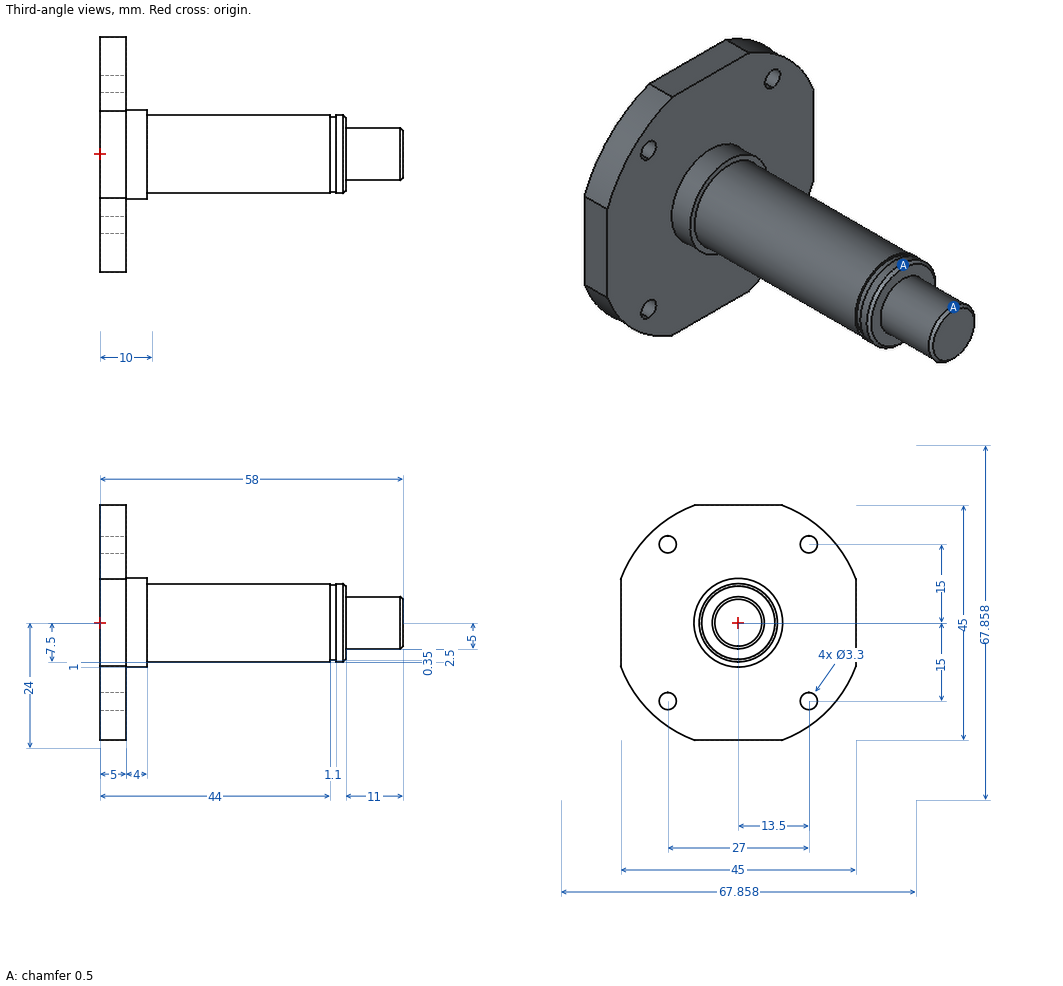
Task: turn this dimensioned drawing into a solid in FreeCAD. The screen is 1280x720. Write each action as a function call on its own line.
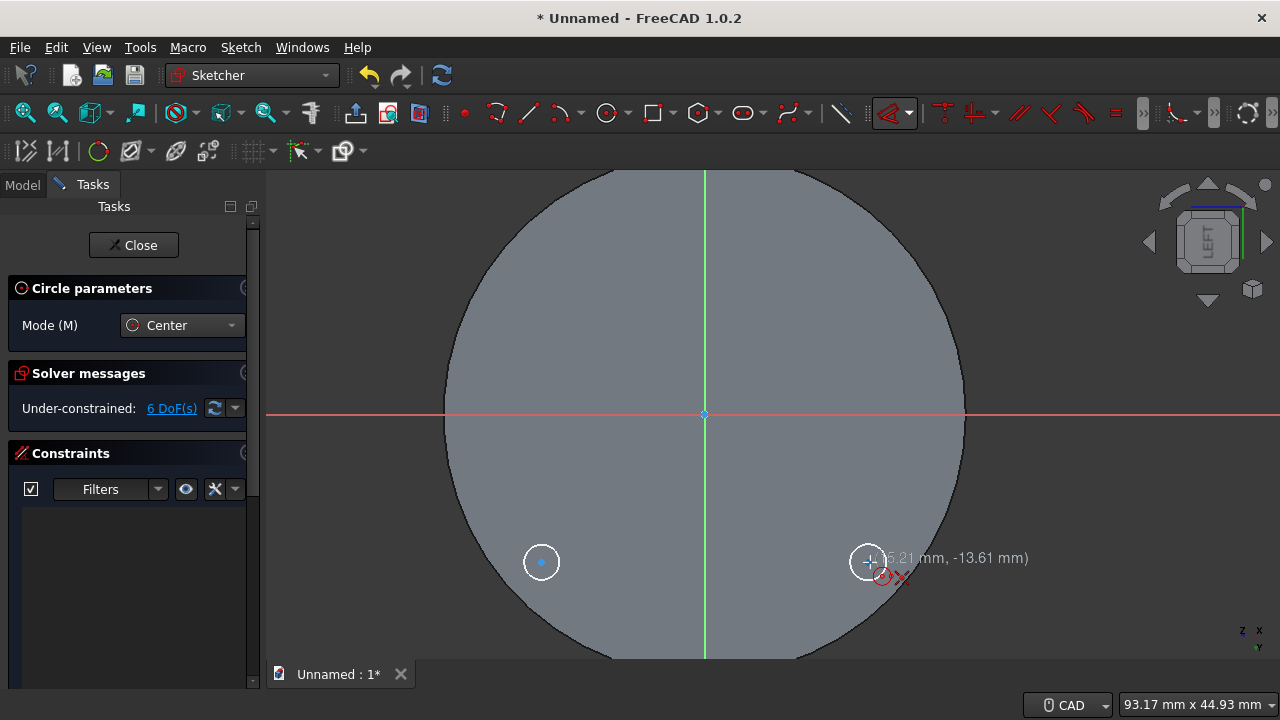
scroll(868, 268, up, 2)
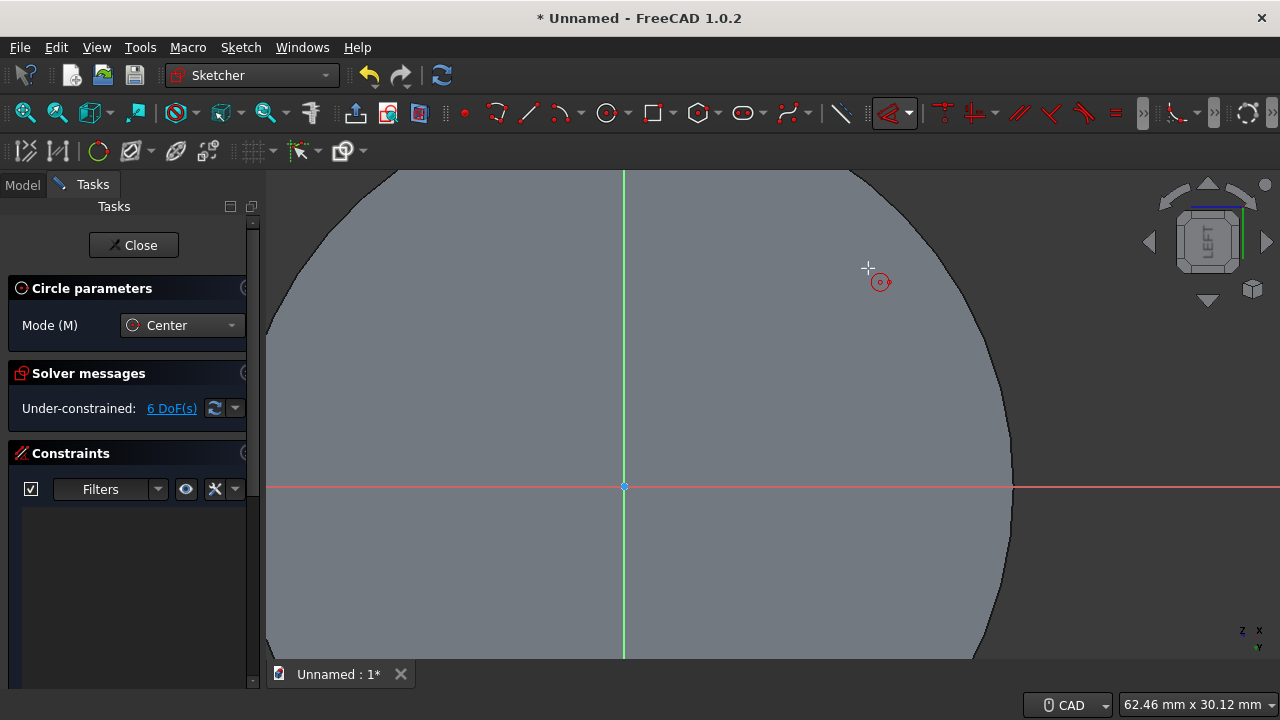
click(868, 268)
click(887, 249)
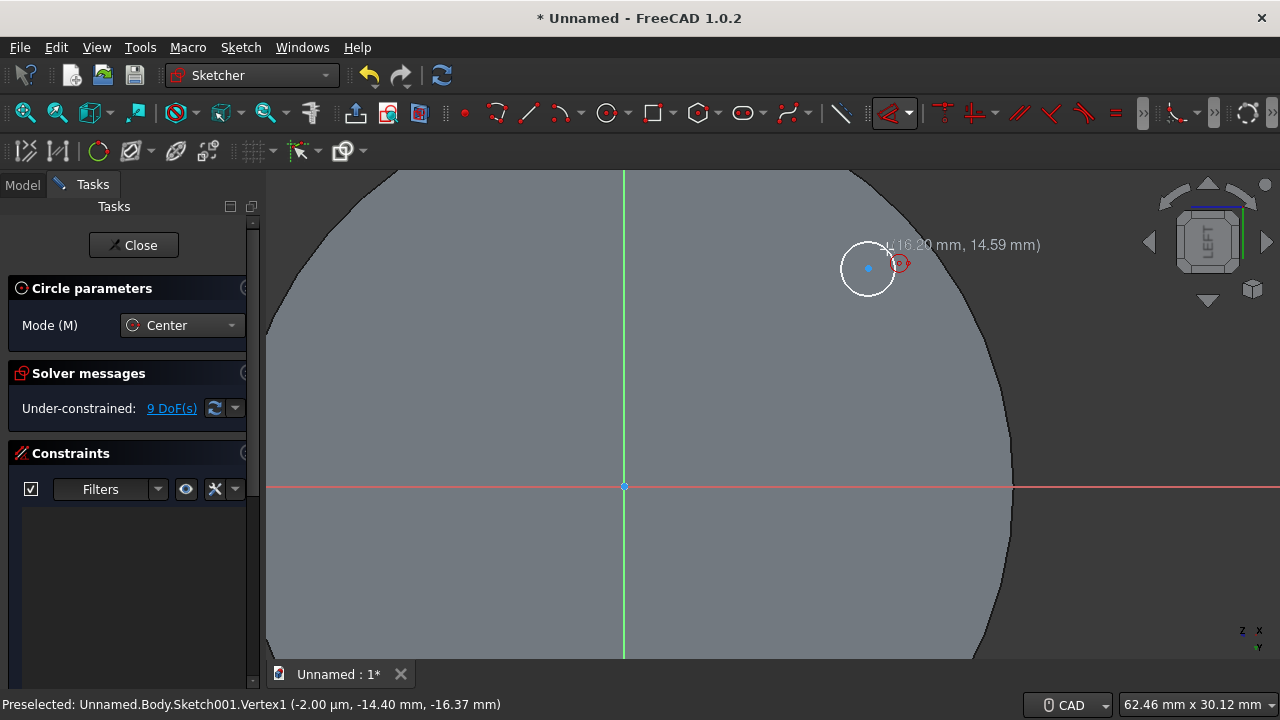
click(381, 268)
click(399, 249)
key(Escape)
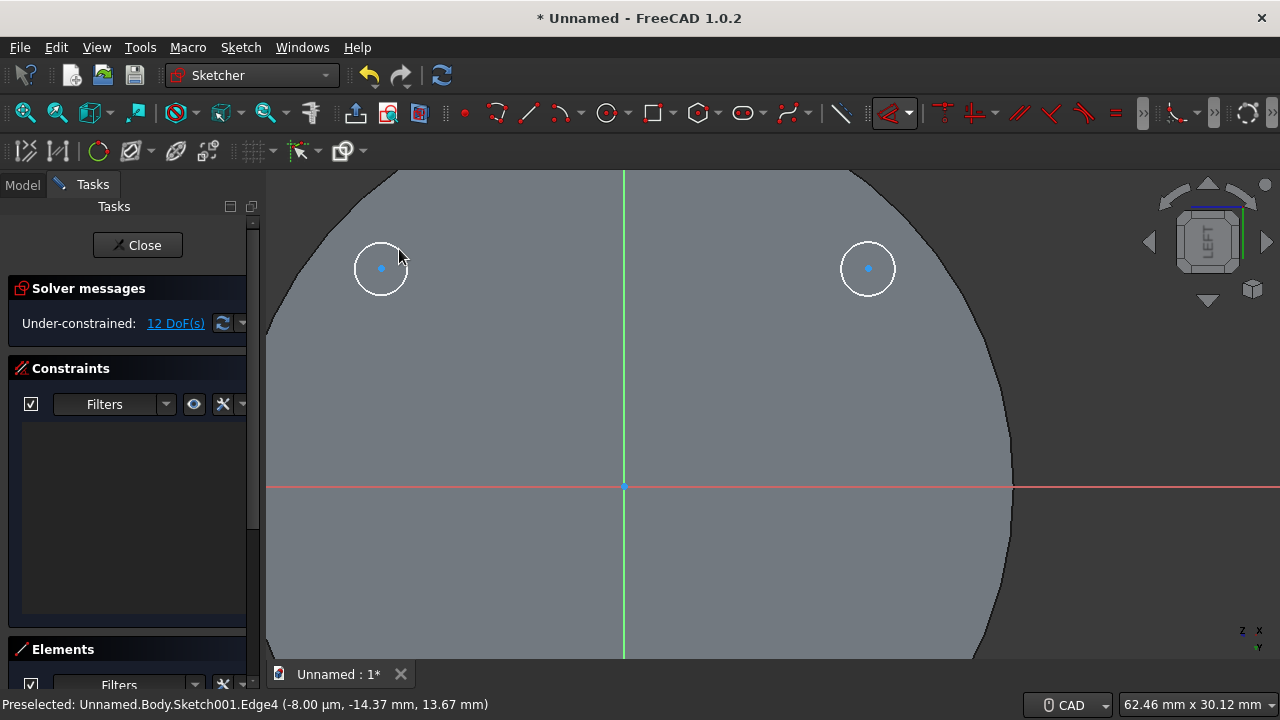
scroll(868, 267, down, 2)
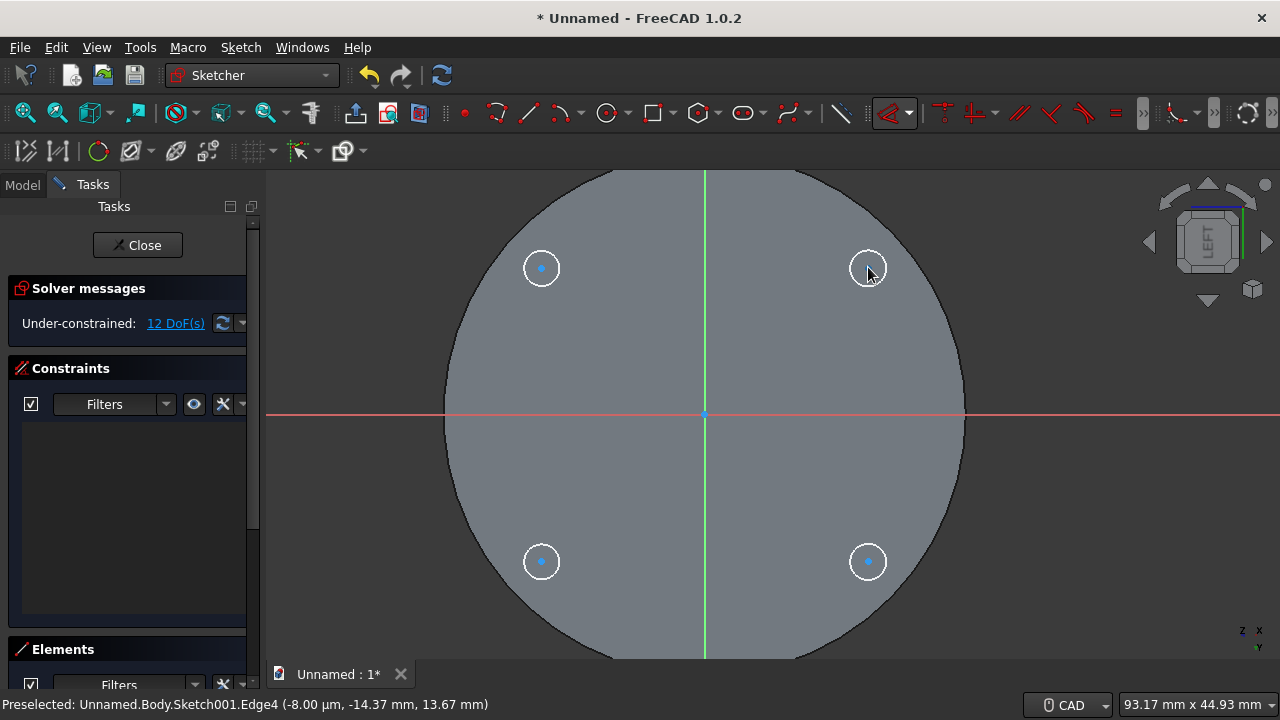
click(881, 549)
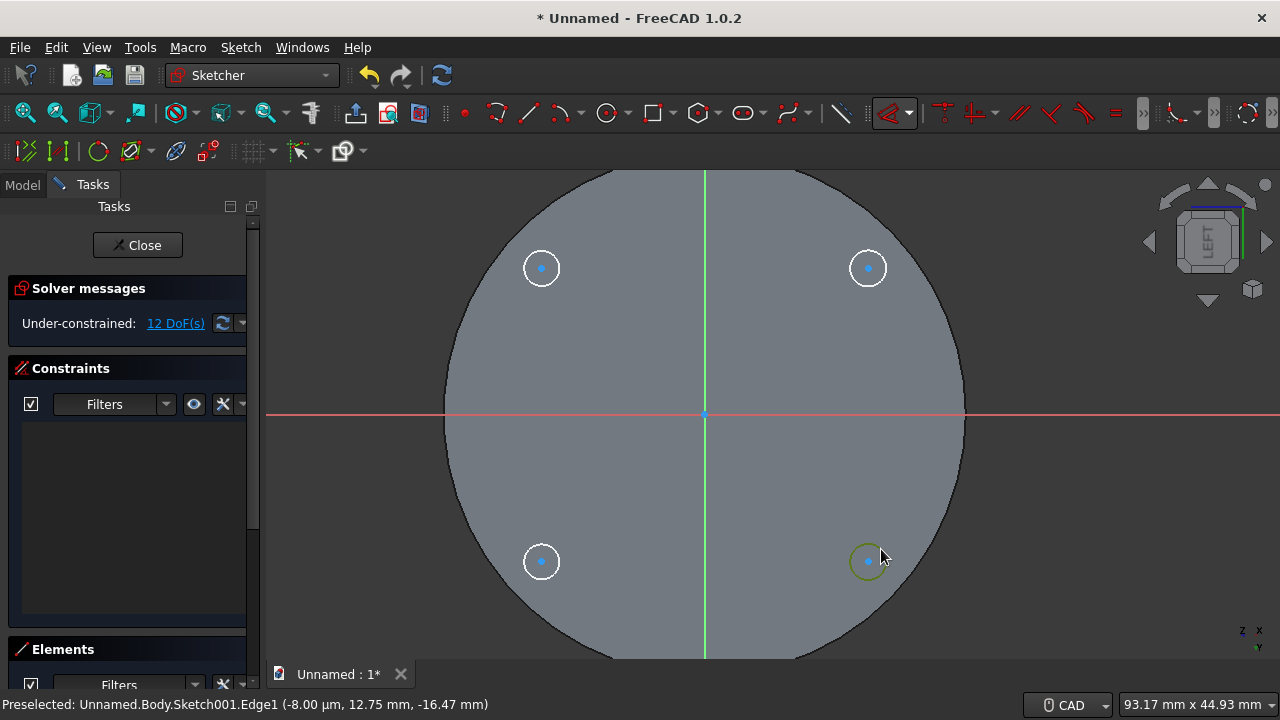
click(554, 549)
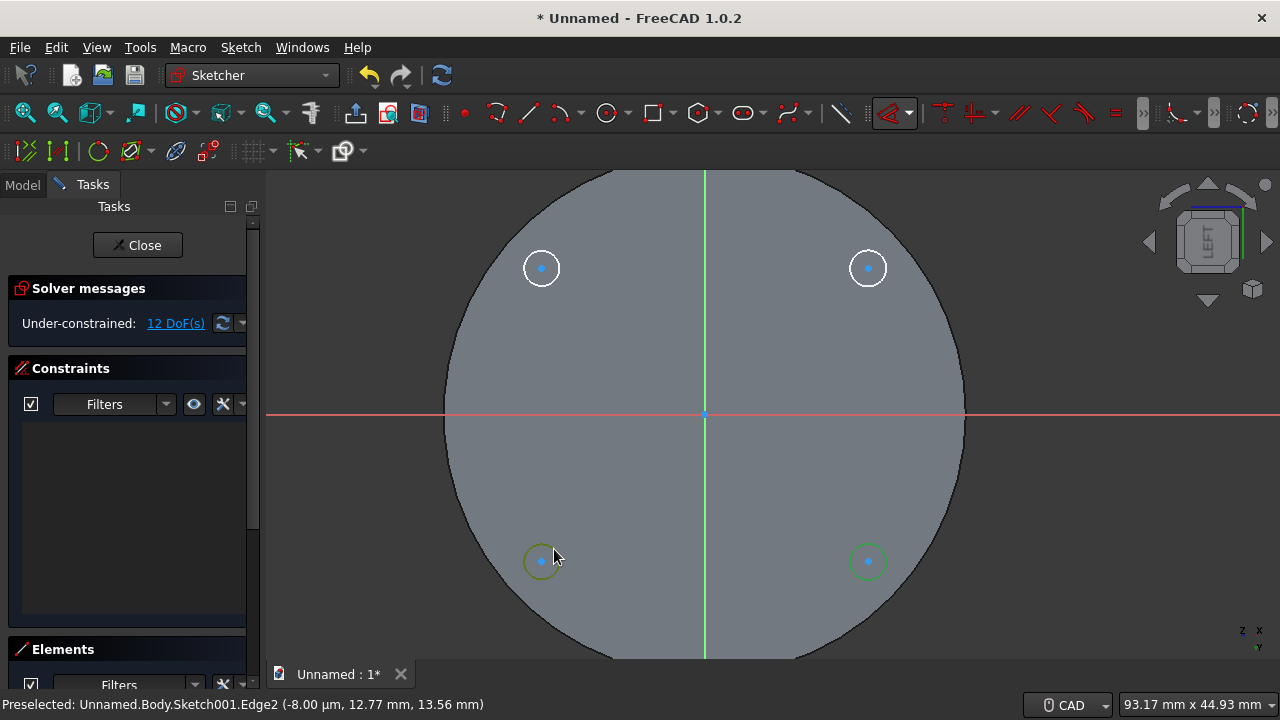
click(881, 256)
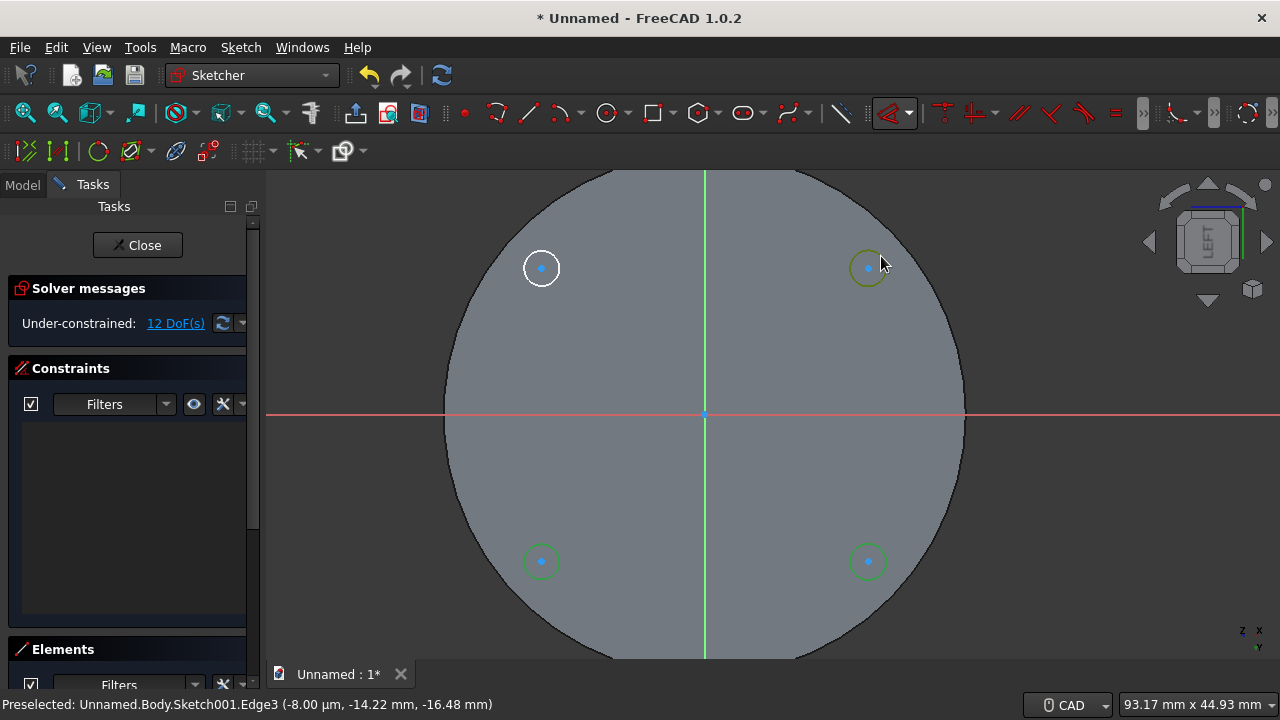
click(554, 256)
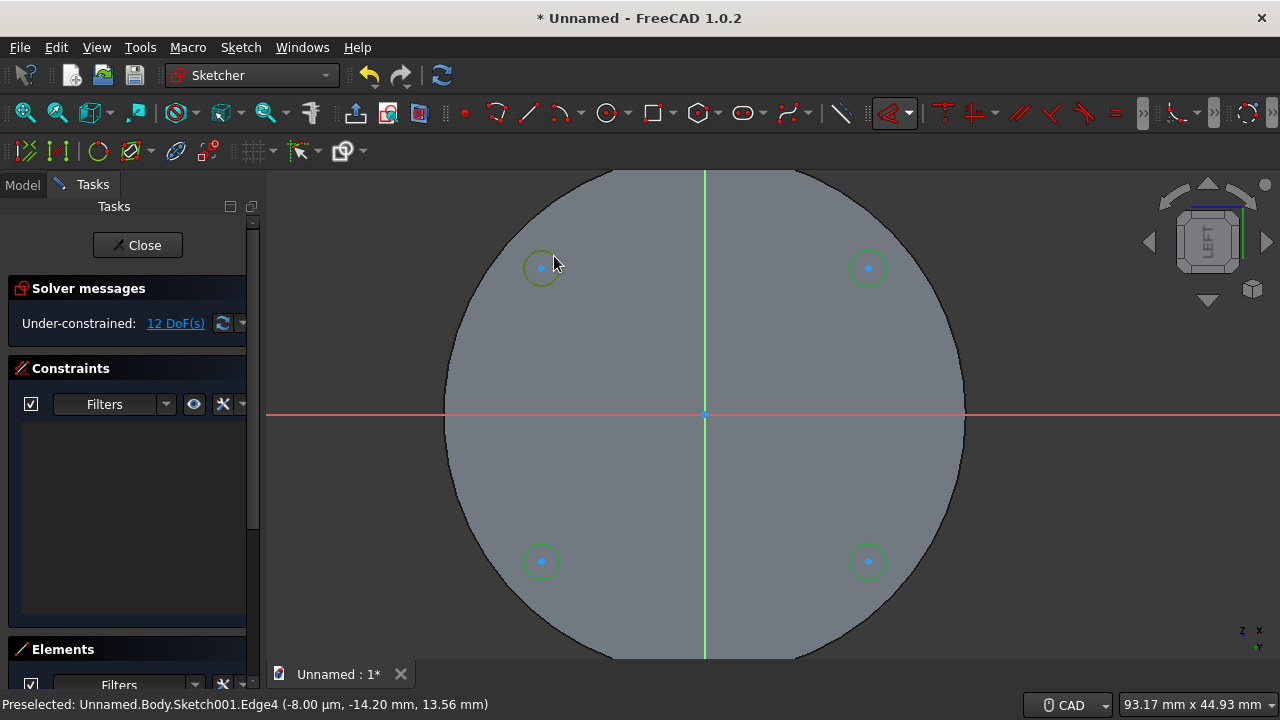
click(1116, 114)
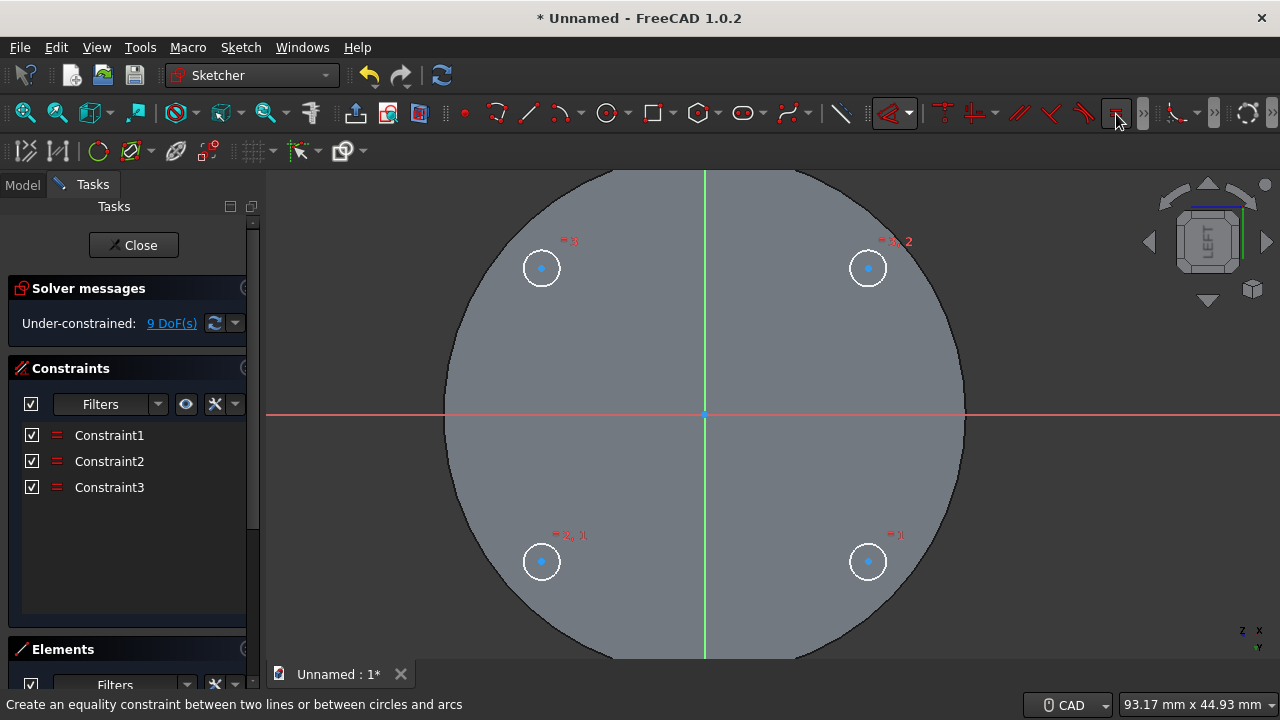
click(868, 562)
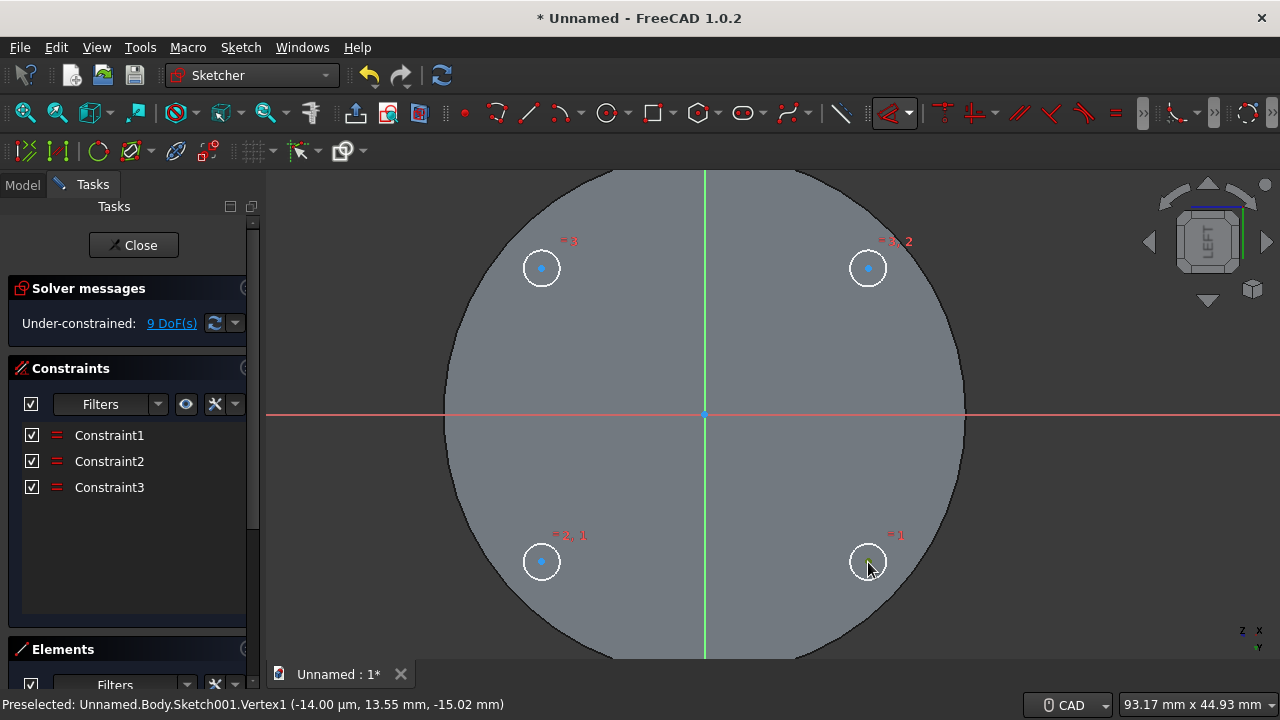
click(542, 562)